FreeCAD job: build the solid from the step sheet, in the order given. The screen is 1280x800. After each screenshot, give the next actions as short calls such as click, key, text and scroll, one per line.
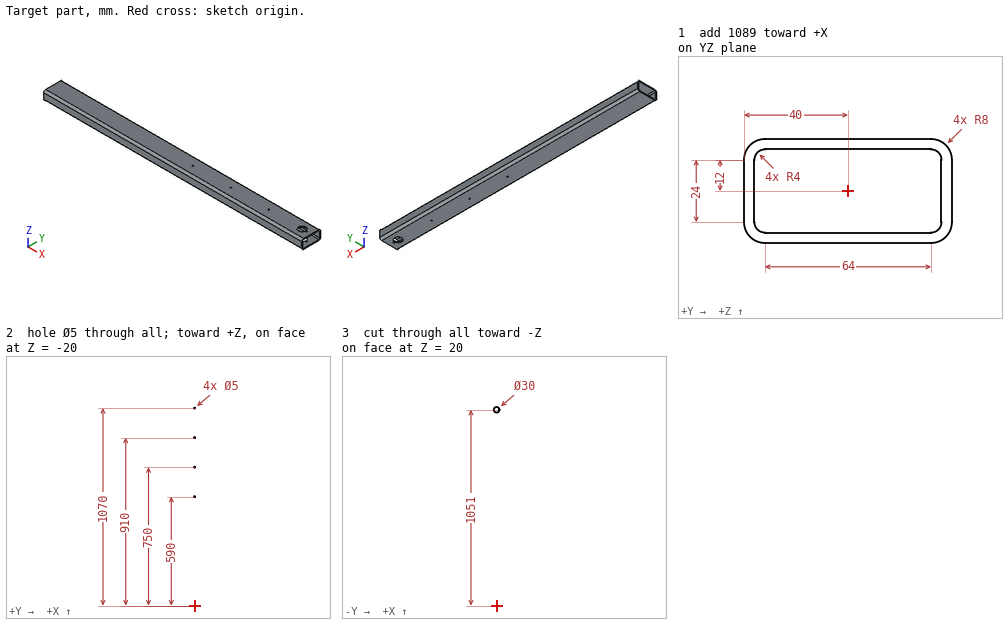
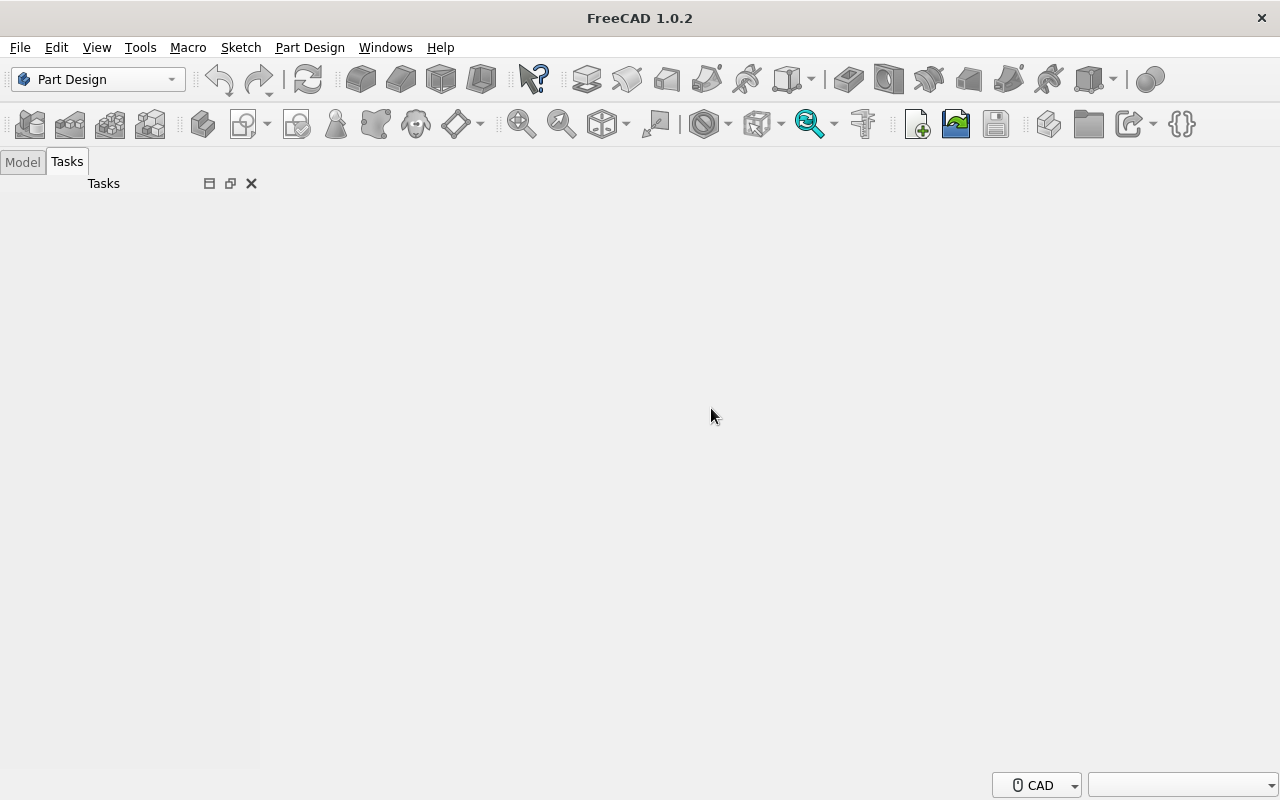
click(916, 124)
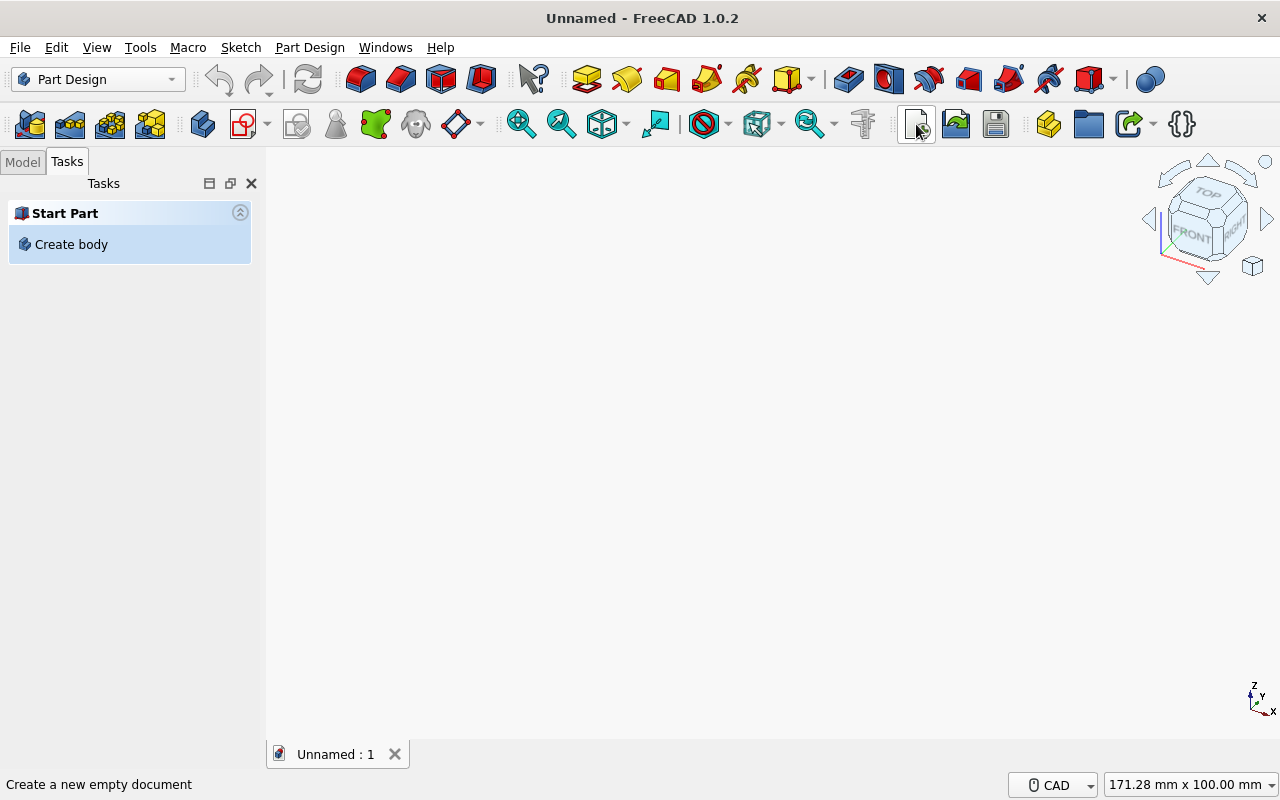
click(244, 124)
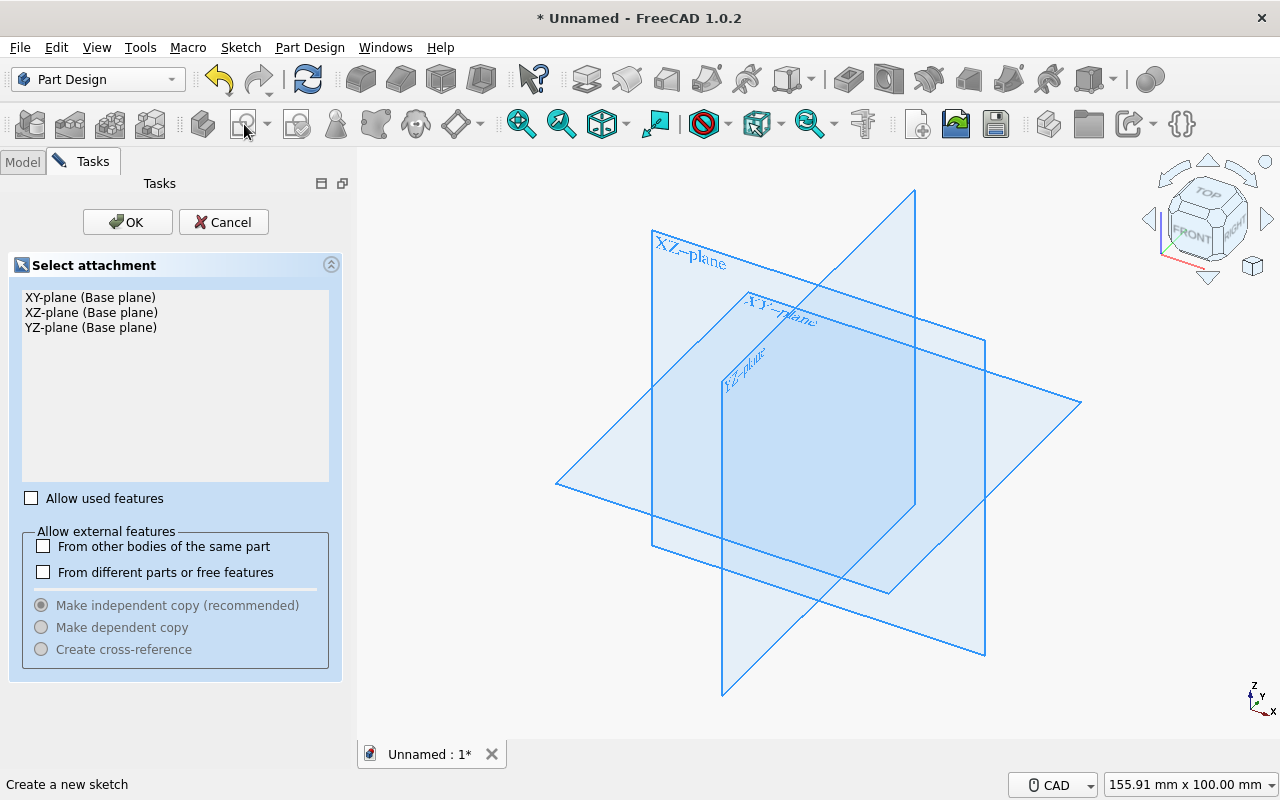
click(82, 328)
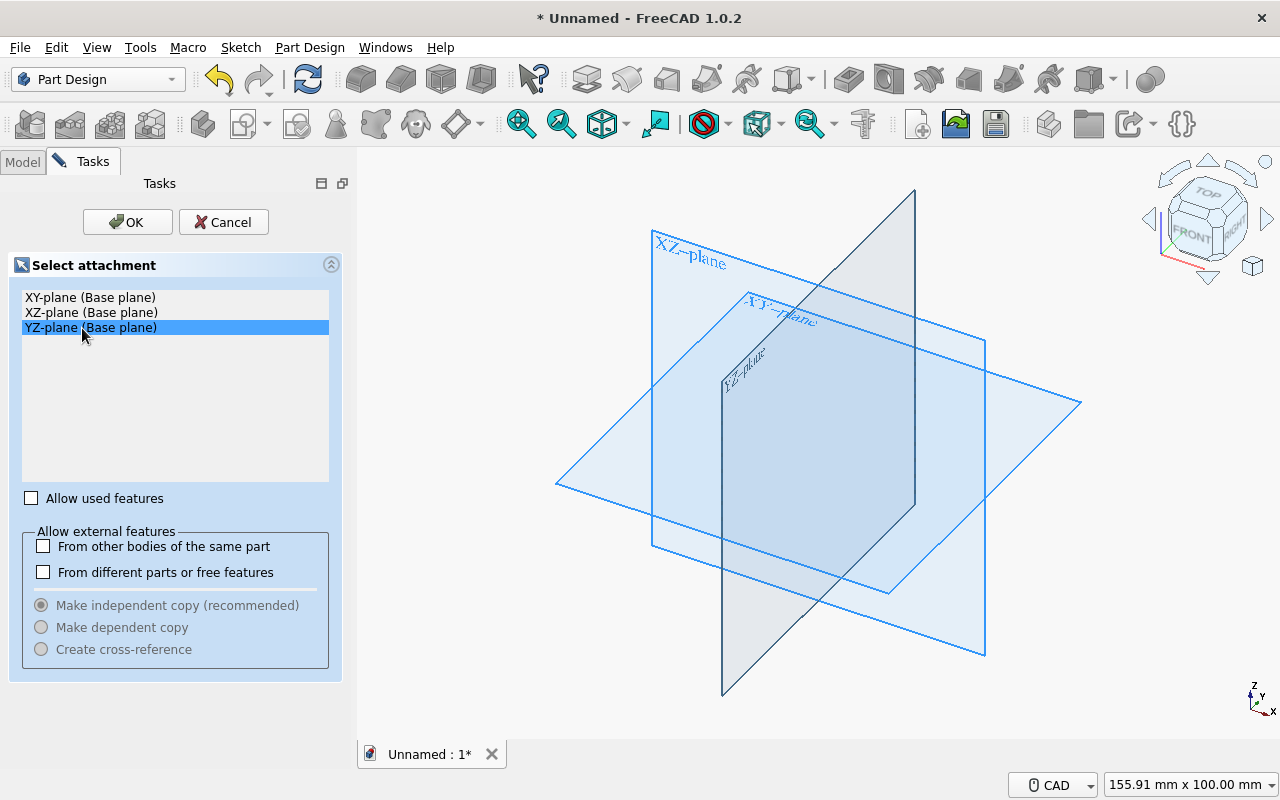
click(128, 222)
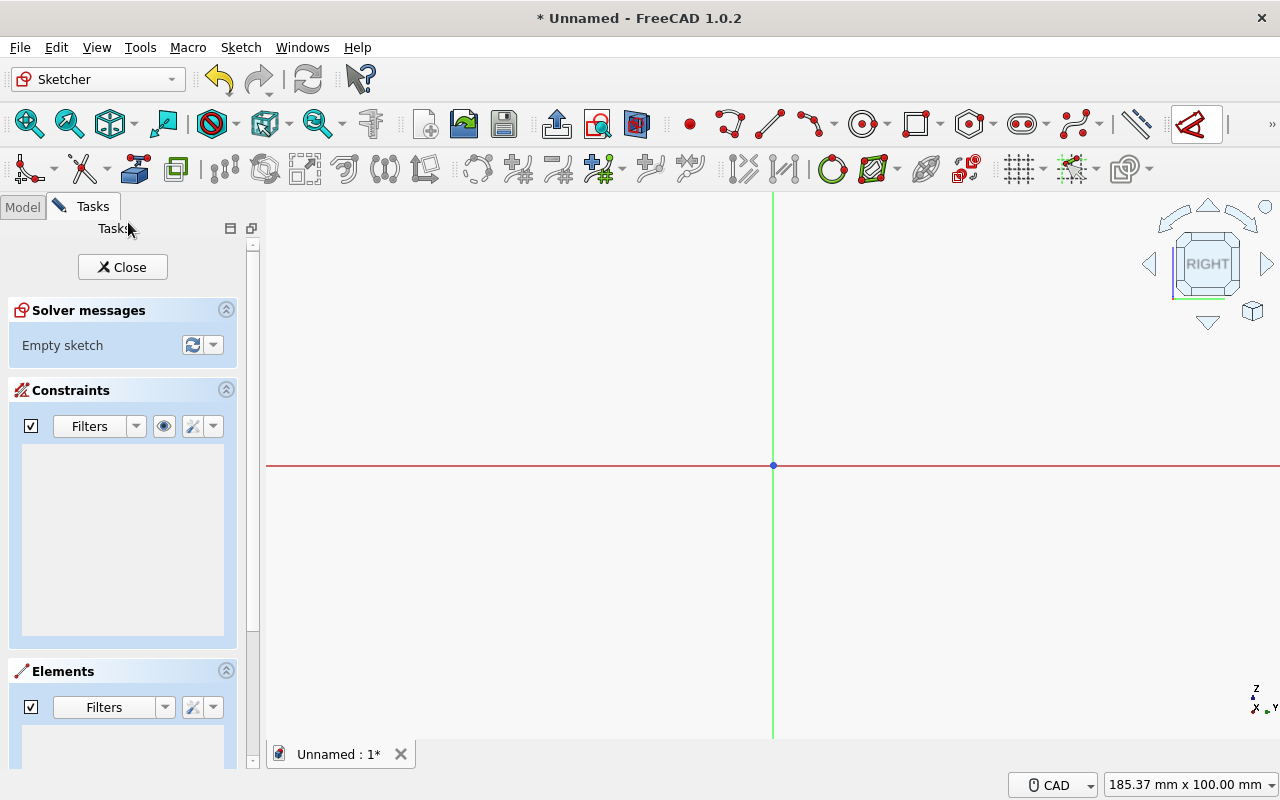
click(770, 124)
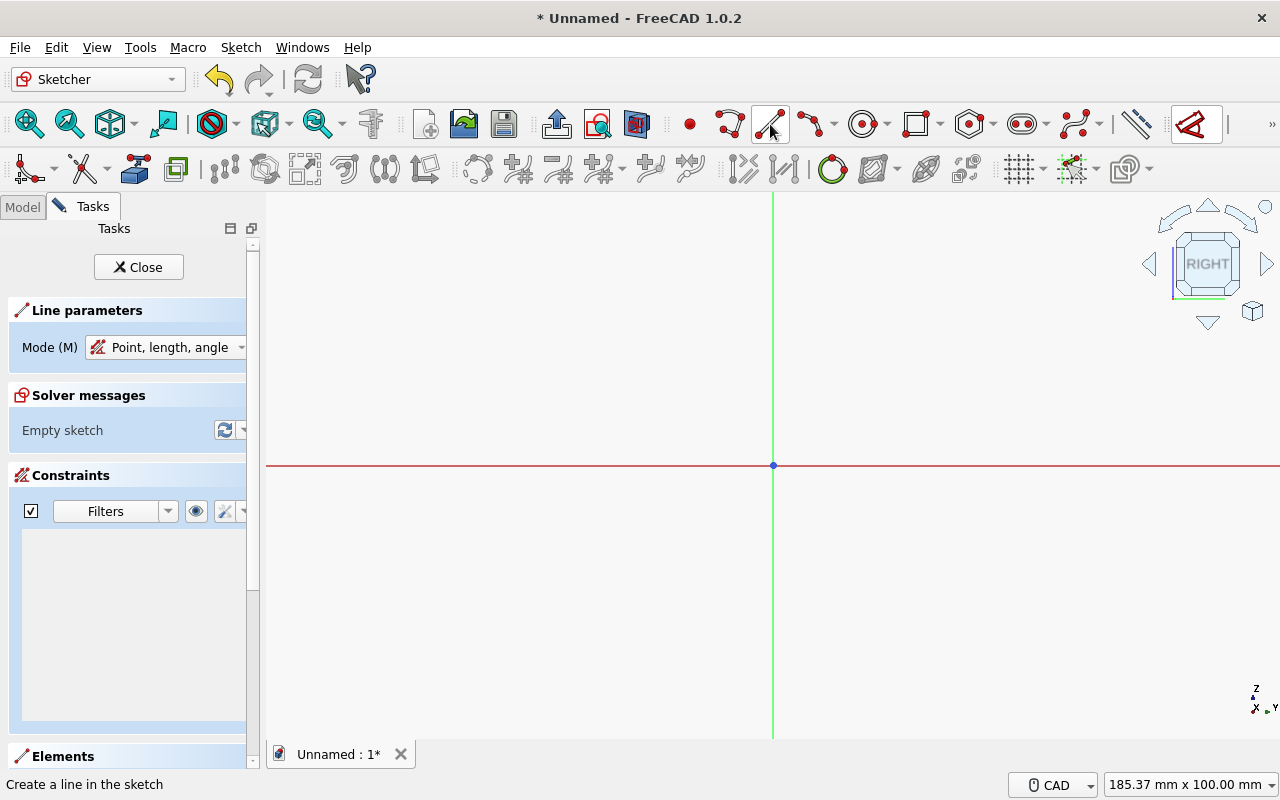
click(554, 400)
click(554, 531)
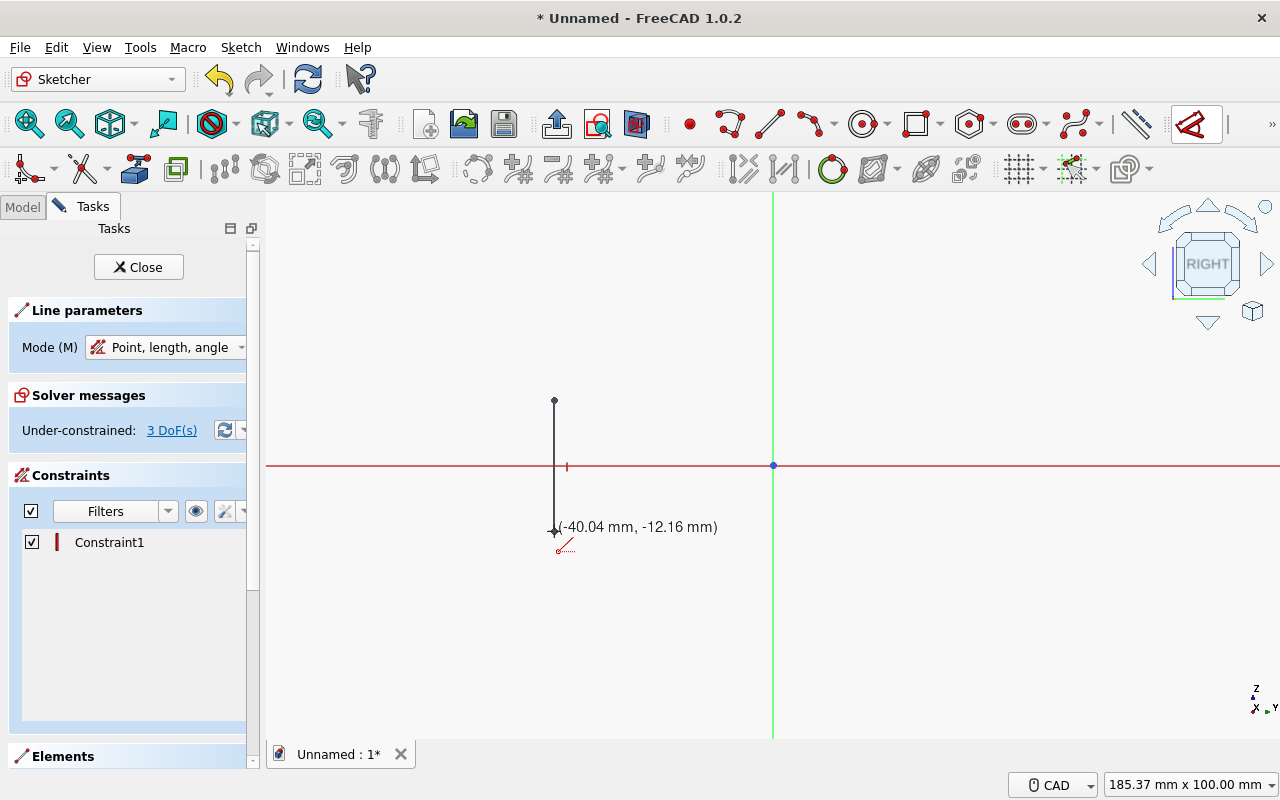
click(598, 575)
click(948, 575)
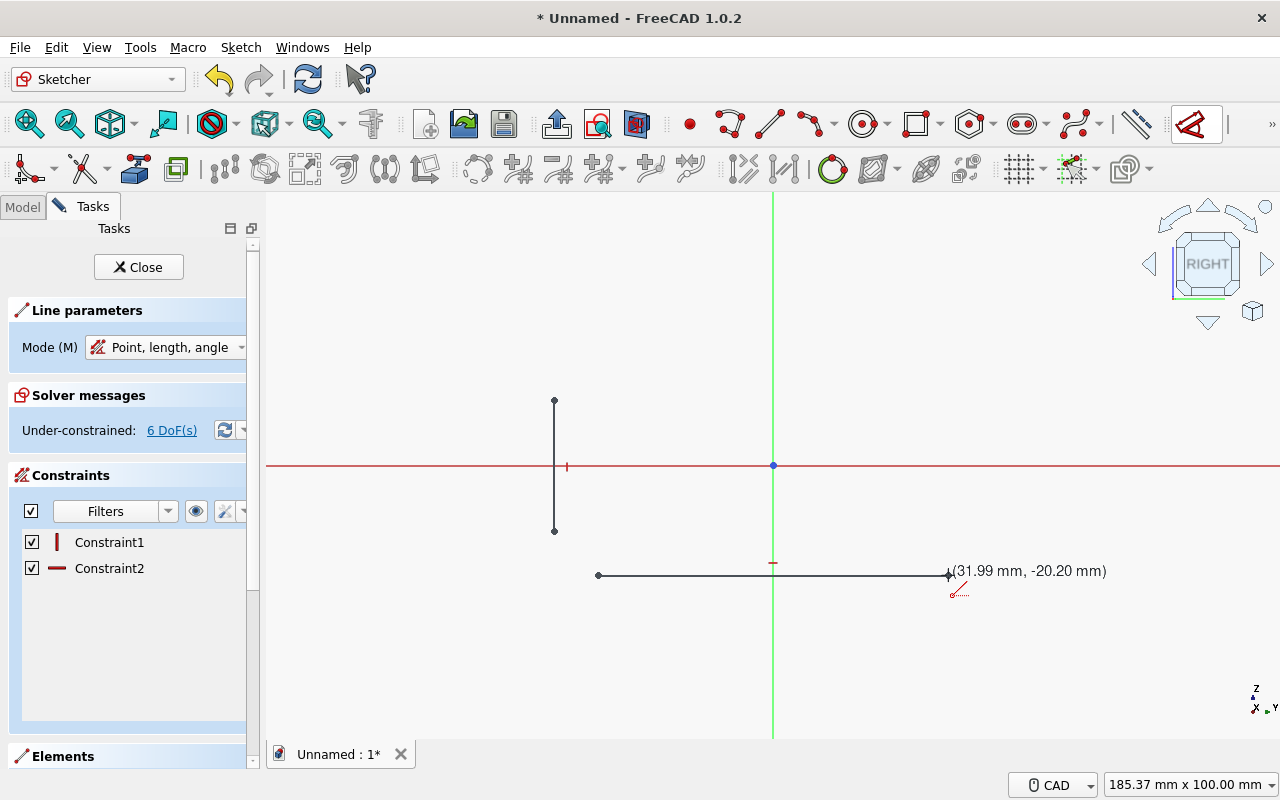
click(992, 531)
click(992, 400)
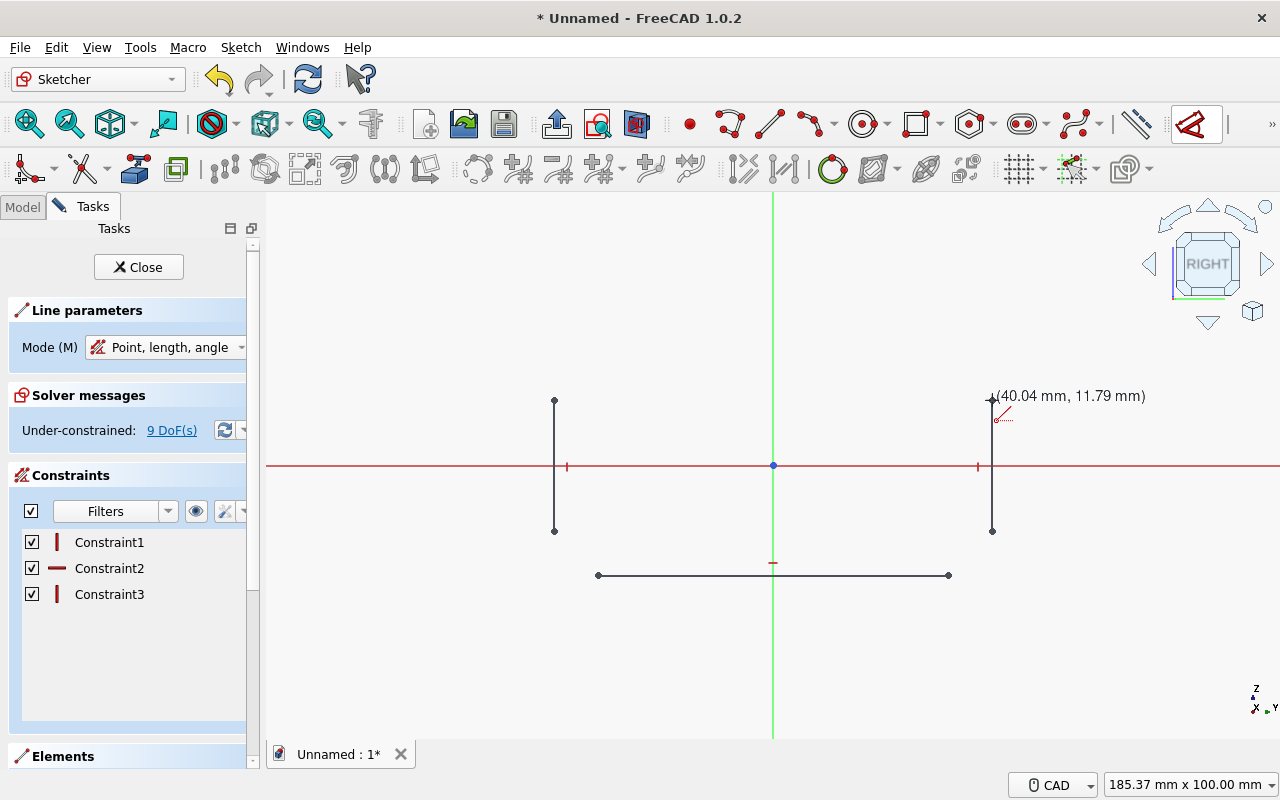
click(948, 356)
click(598, 356)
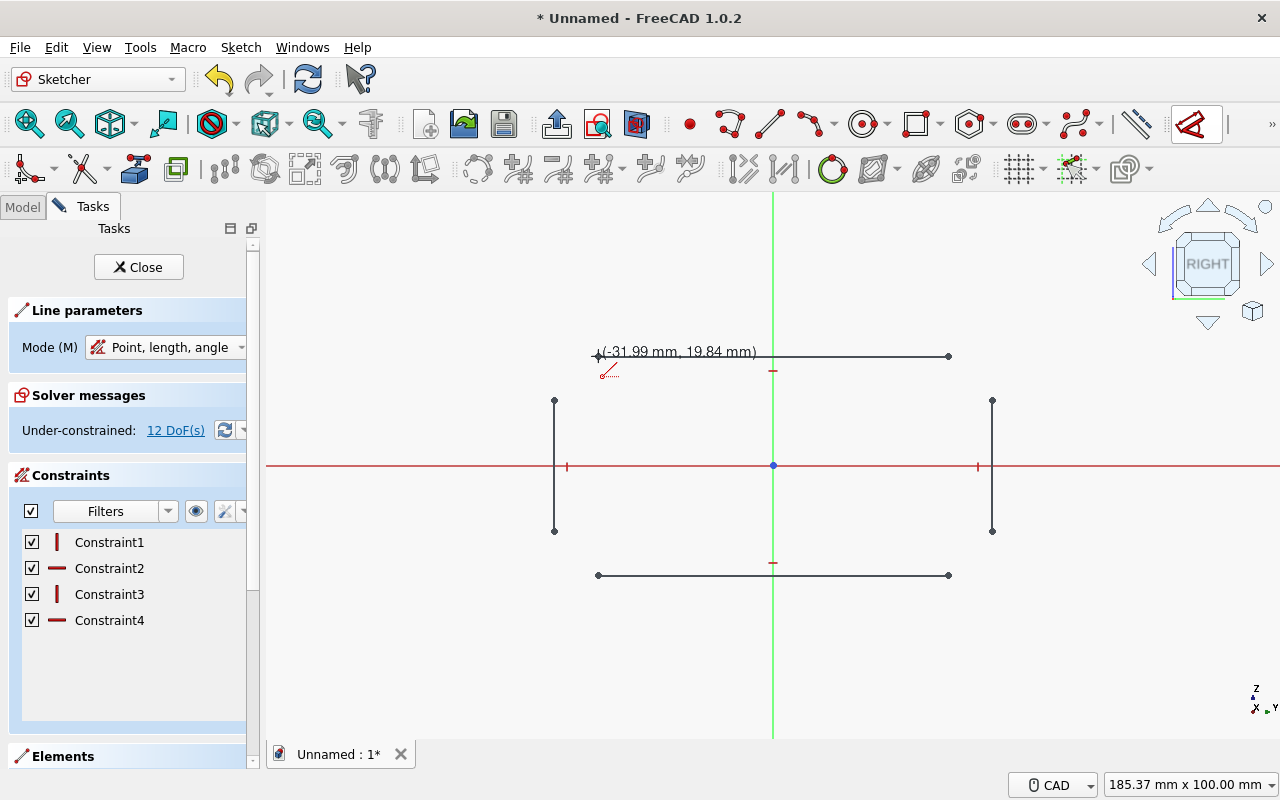
click(810, 124)